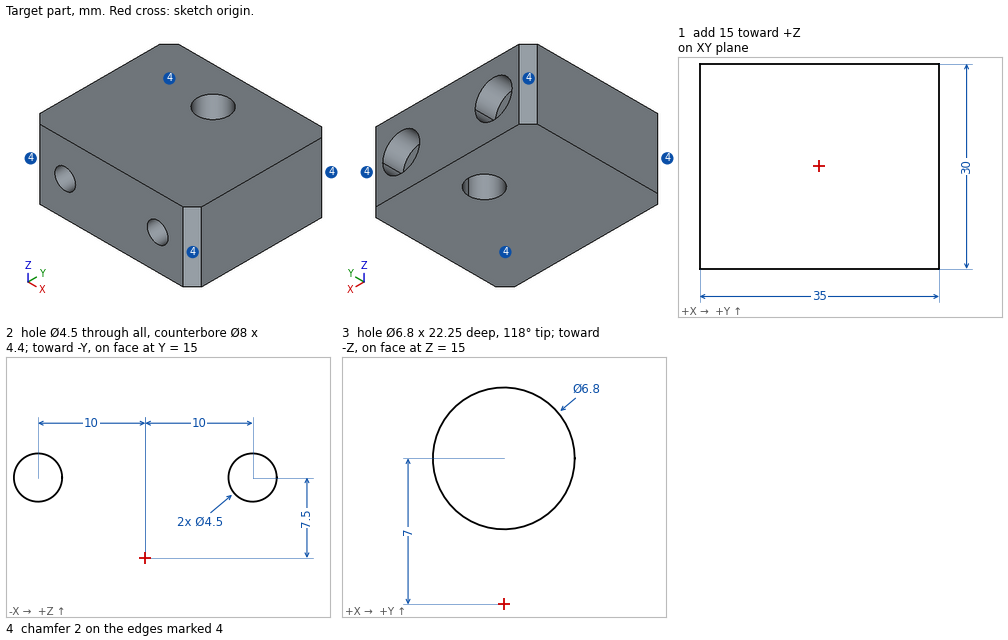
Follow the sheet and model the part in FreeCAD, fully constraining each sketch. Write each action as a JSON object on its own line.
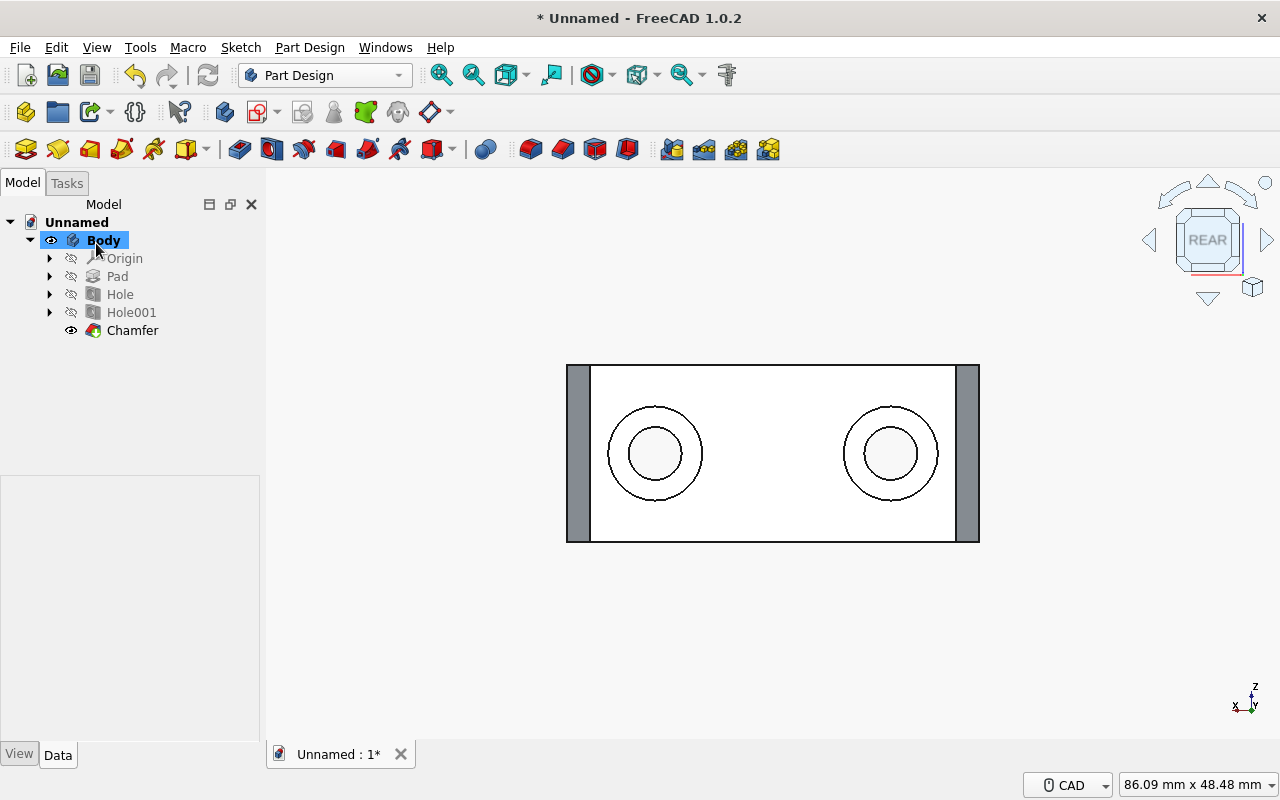
{"action": "key", "text": "0"}